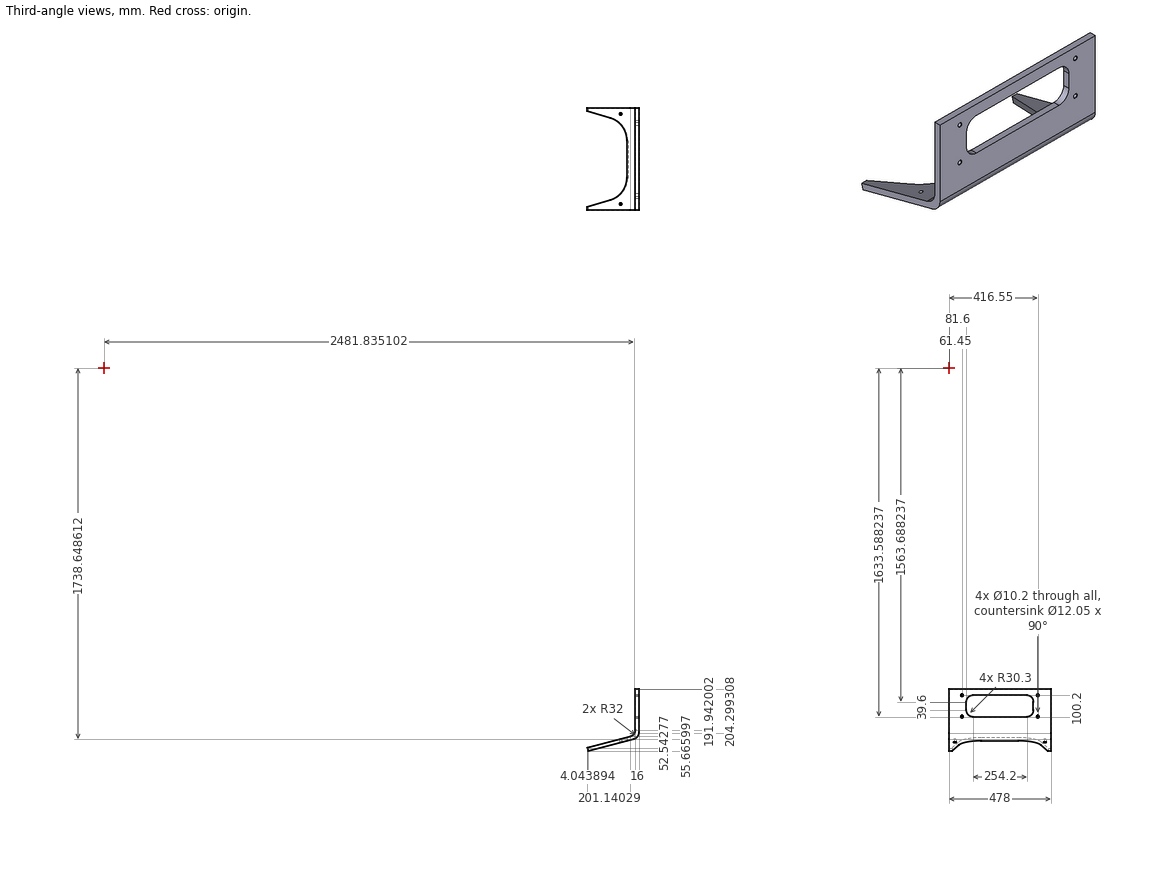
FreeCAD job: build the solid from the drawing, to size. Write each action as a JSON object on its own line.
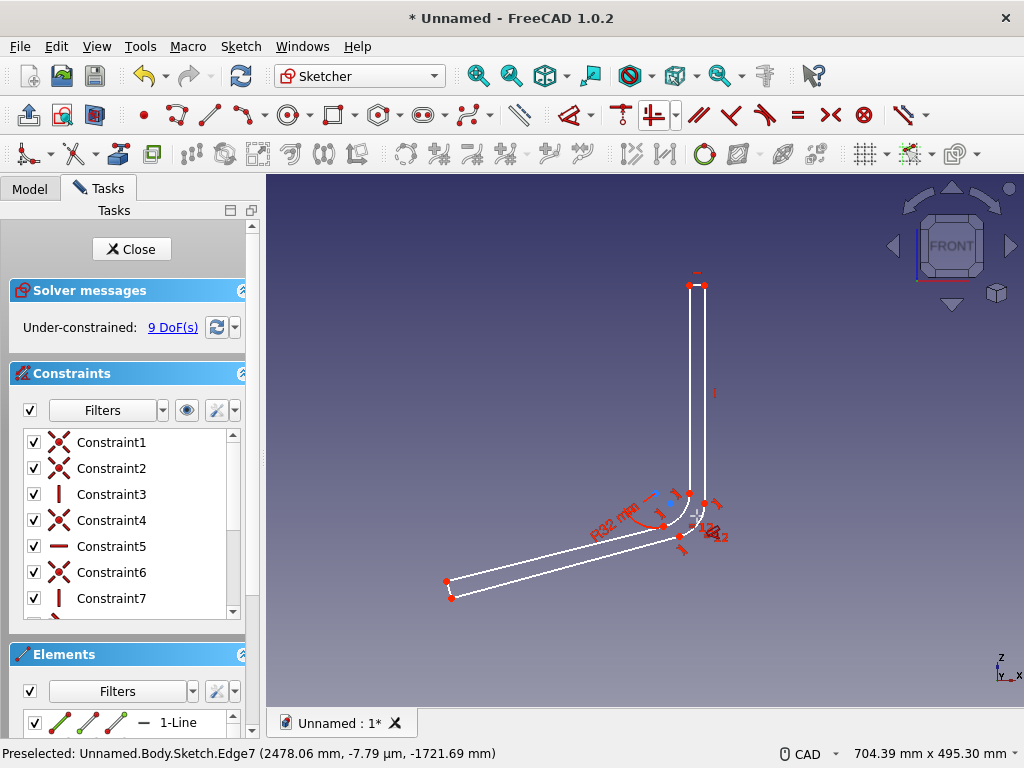
{"action": "scroll", "coordinate": [694, 285], "scroll_direction": "up", "scroll_amount": 6}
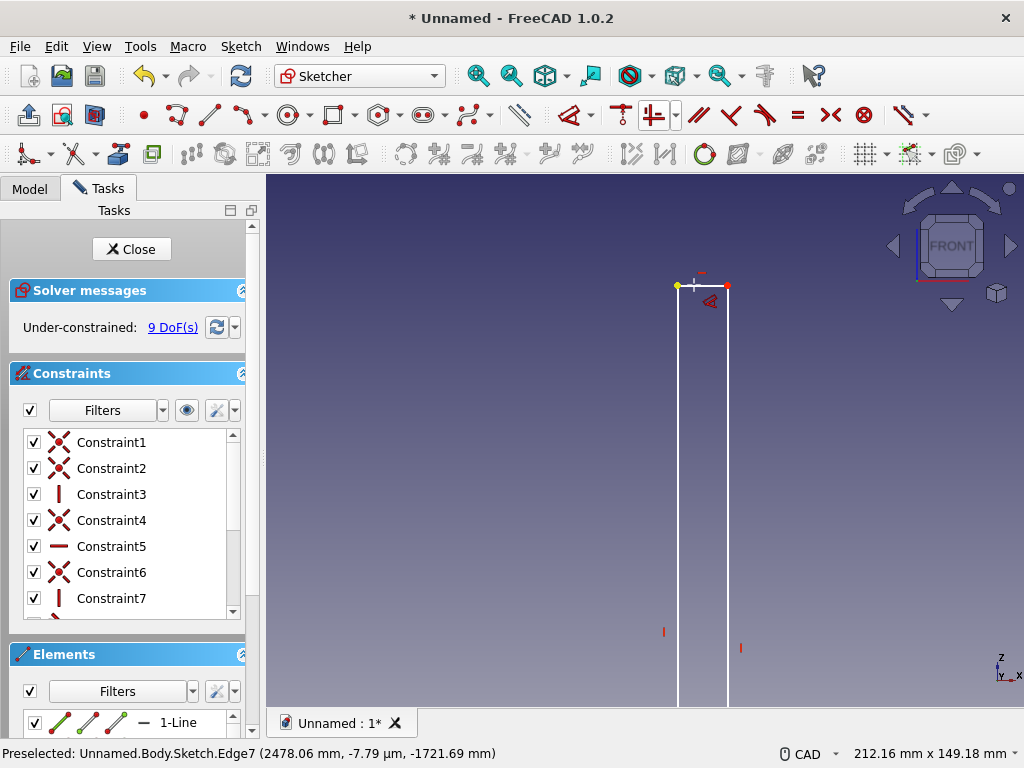
{"action": "left_click", "coordinate": [693, 286]}
{"action": "left_click", "coordinate": [703, 252]}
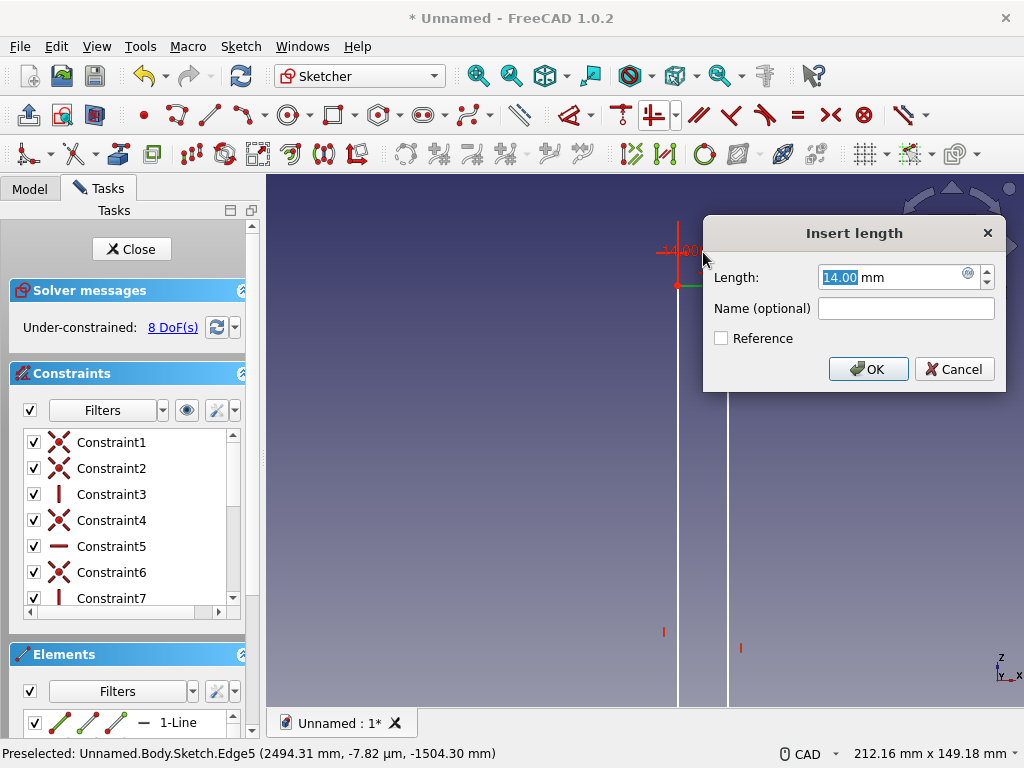
{"action": "type", "text": "16"}
{"action": "key", "text": "Return"}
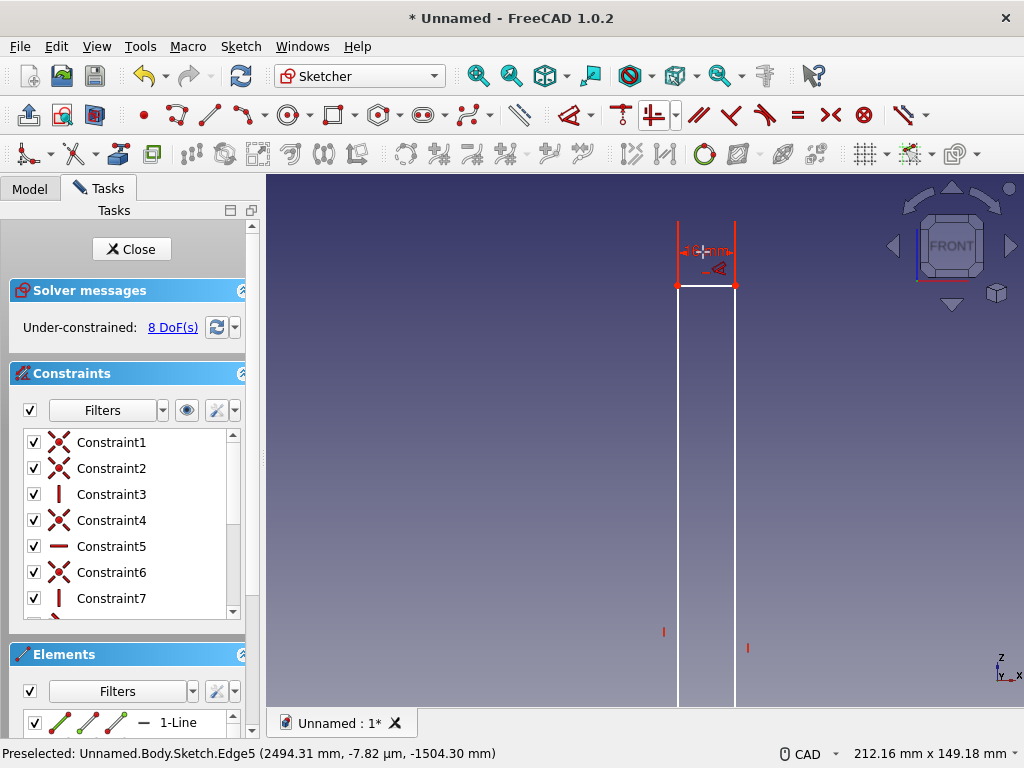
{"action": "scroll", "coordinate": [694, 285], "scroll_direction": "down", "scroll_amount": 6}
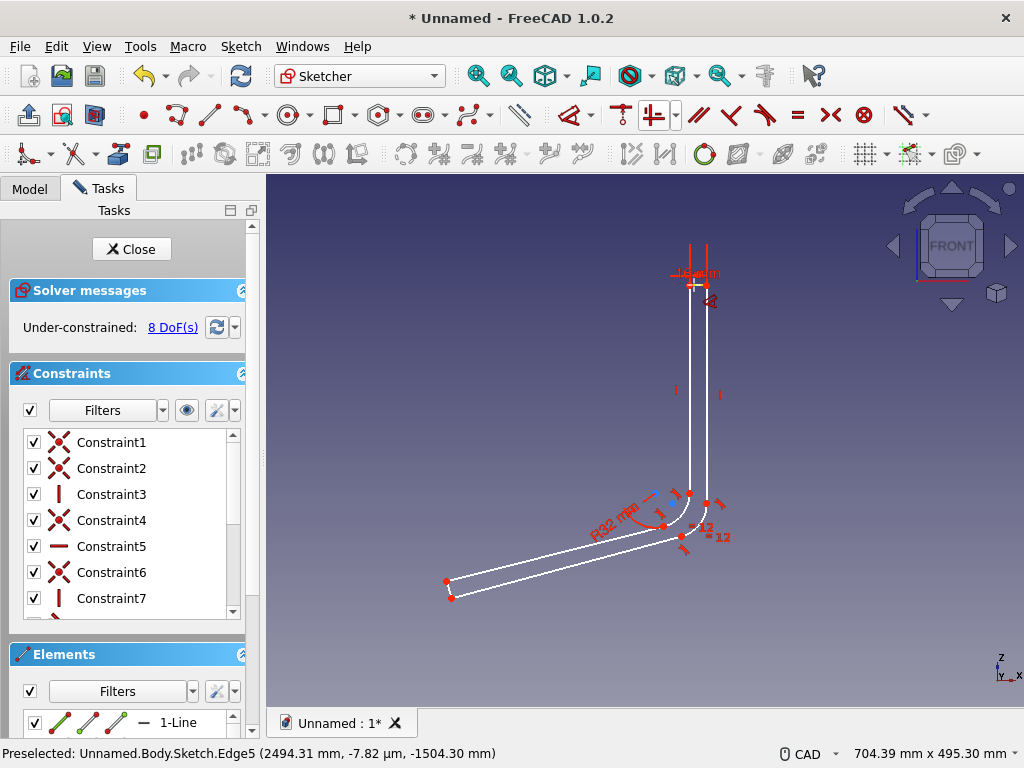
{"action": "scroll", "coordinate": [450, 593], "scroll_direction": "up", "scroll_amount": 12}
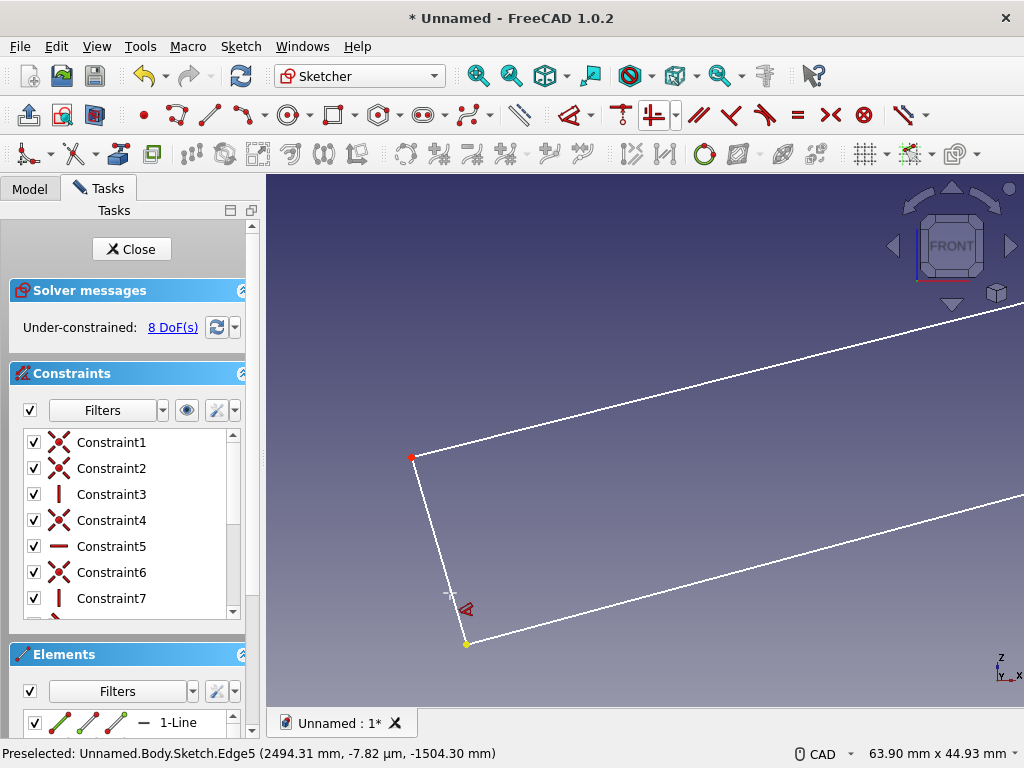
{"action": "left_click", "coordinate": [450, 589]}
{"action": "left_click", "coordinate": [439, 679]}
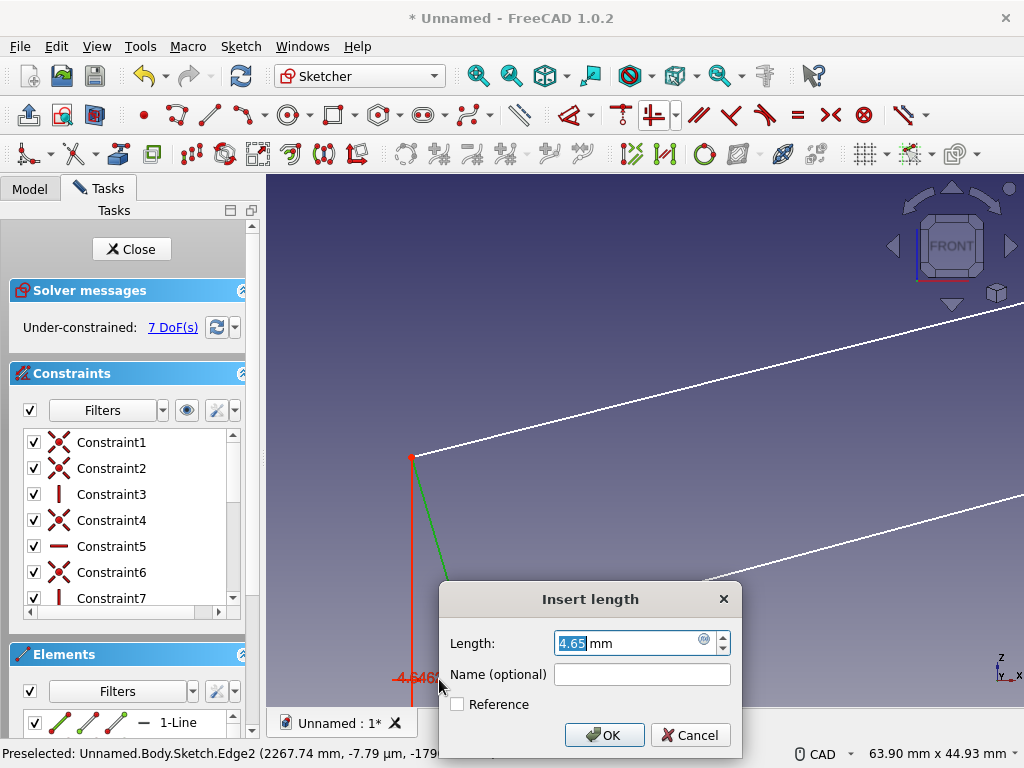
{"action": "type", "text": "4.043894"}
{"action": "key", "text": "Return"}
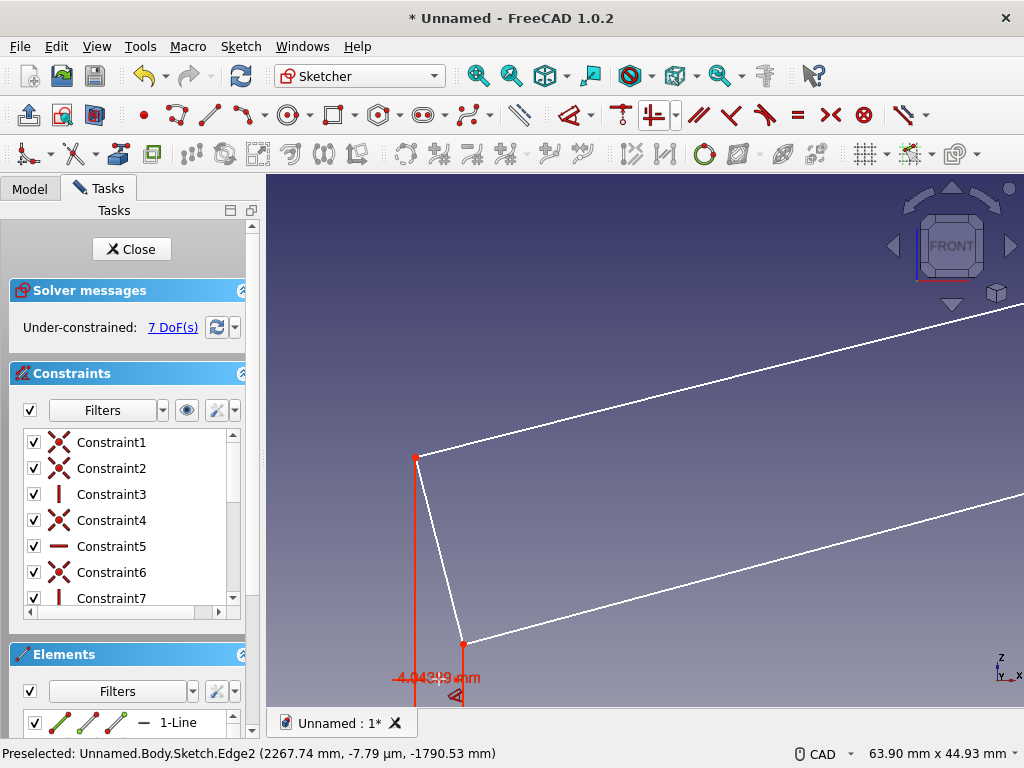
{"action": "scroll", "coordinate": [450, 593], "scroll_direction": "down", "scroll_amount": 12}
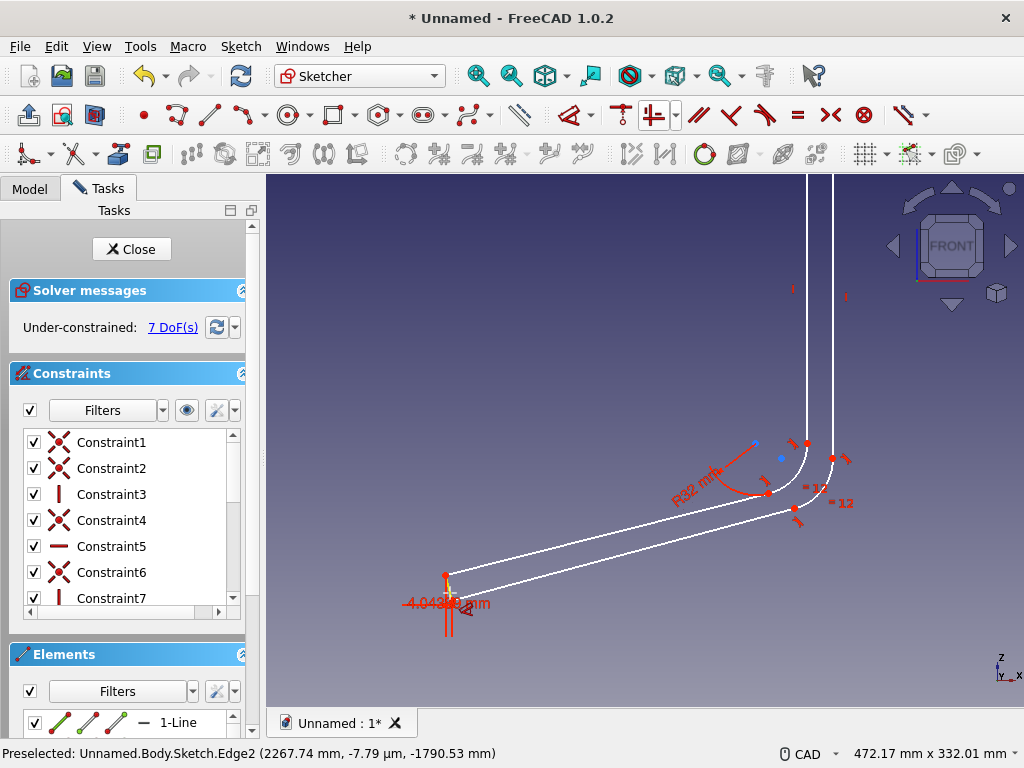
{"action": "left_click", "coordinate": [512, 565]}
{"action": "left_click", "coordinate": [413, 554]}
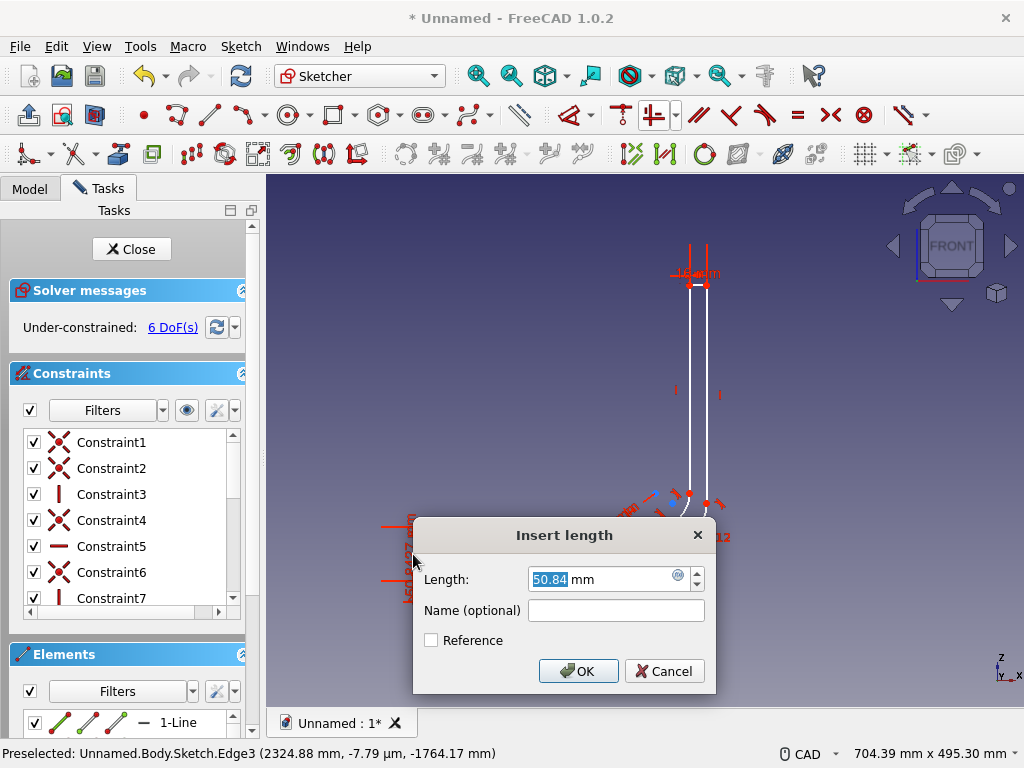
{"action": "type", "text": "52.54277"}
{"action": "key", "text": "Return"}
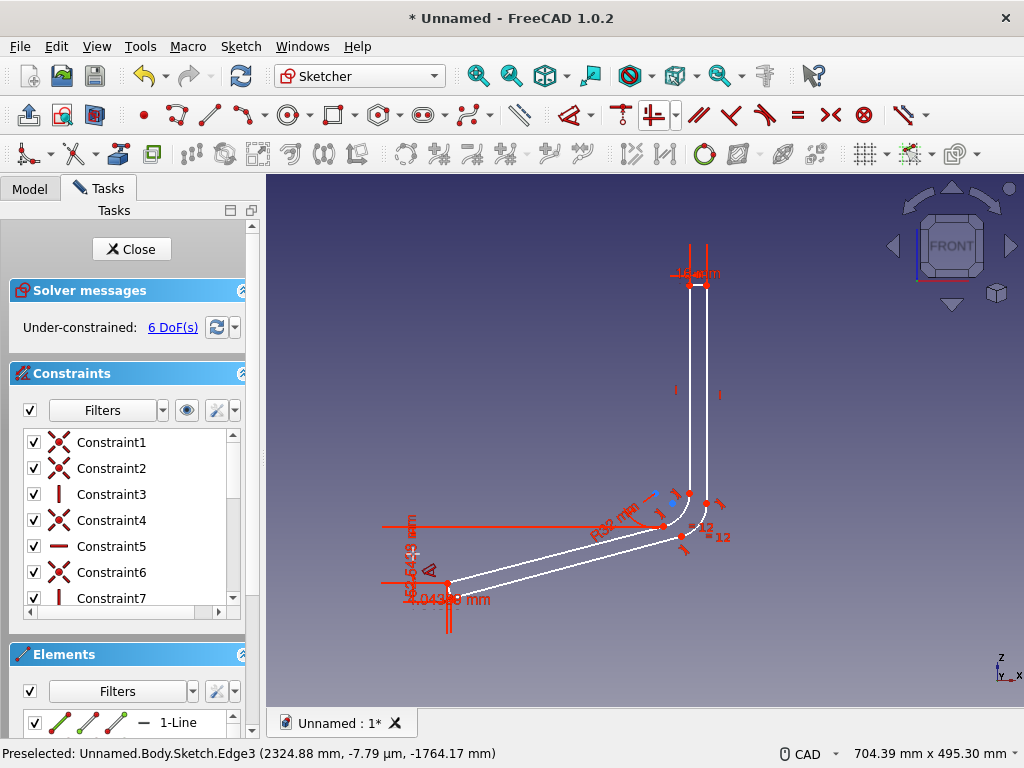
{"action": "left_click", "coordinate": [690, 431]}
{"action": "left_click", "coordinate": [724, 389]}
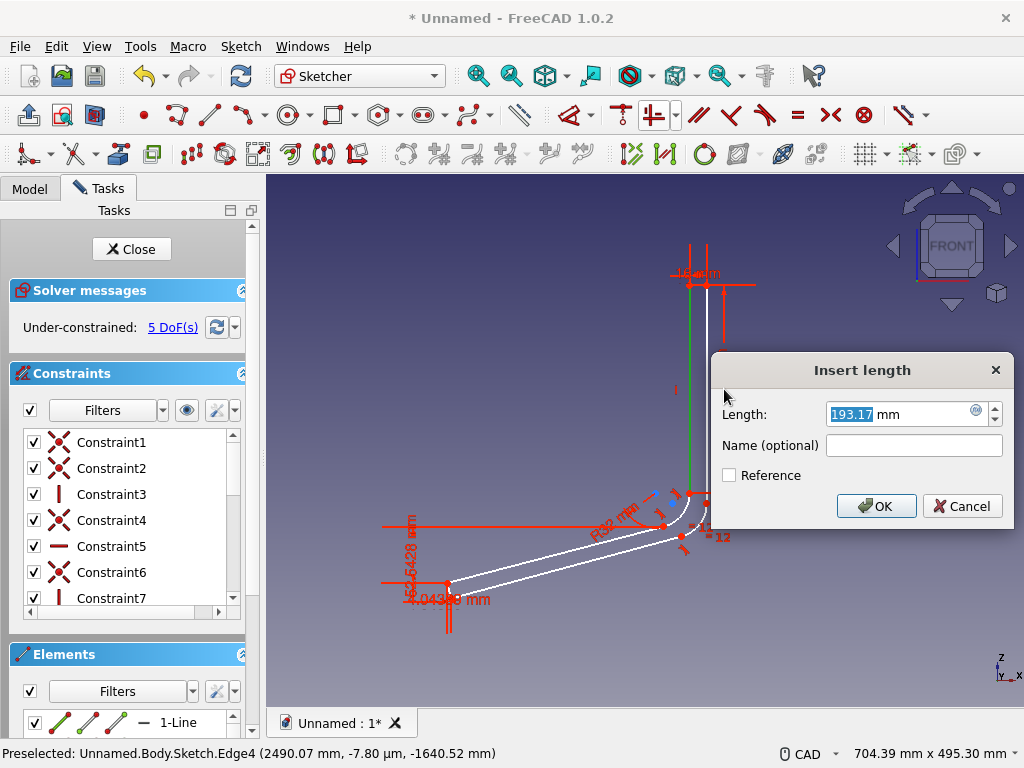
{"action": "type", "text": "191.942002"}
{"action": "key", "text": "Return"}